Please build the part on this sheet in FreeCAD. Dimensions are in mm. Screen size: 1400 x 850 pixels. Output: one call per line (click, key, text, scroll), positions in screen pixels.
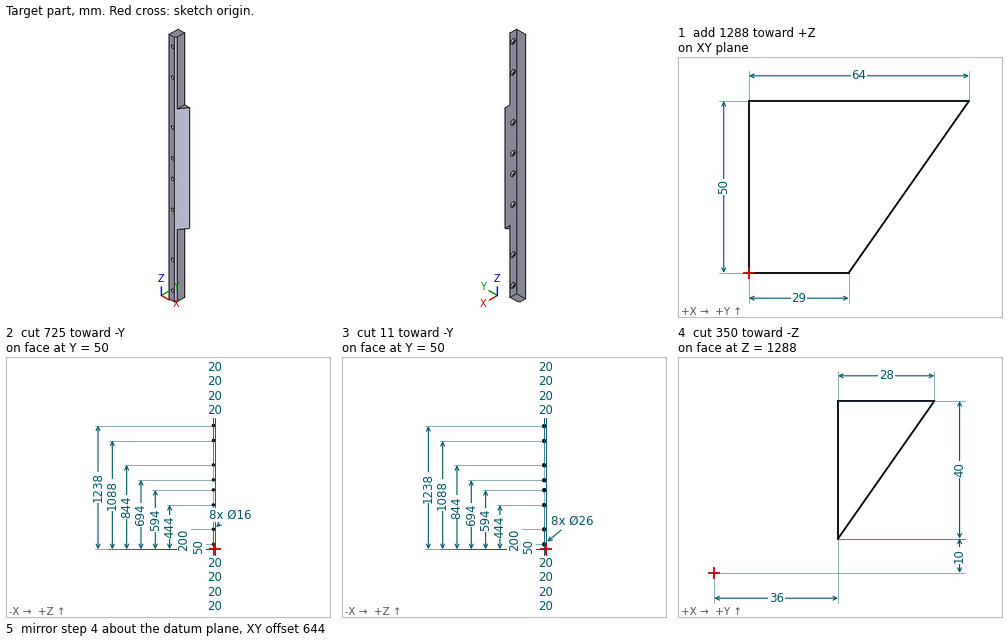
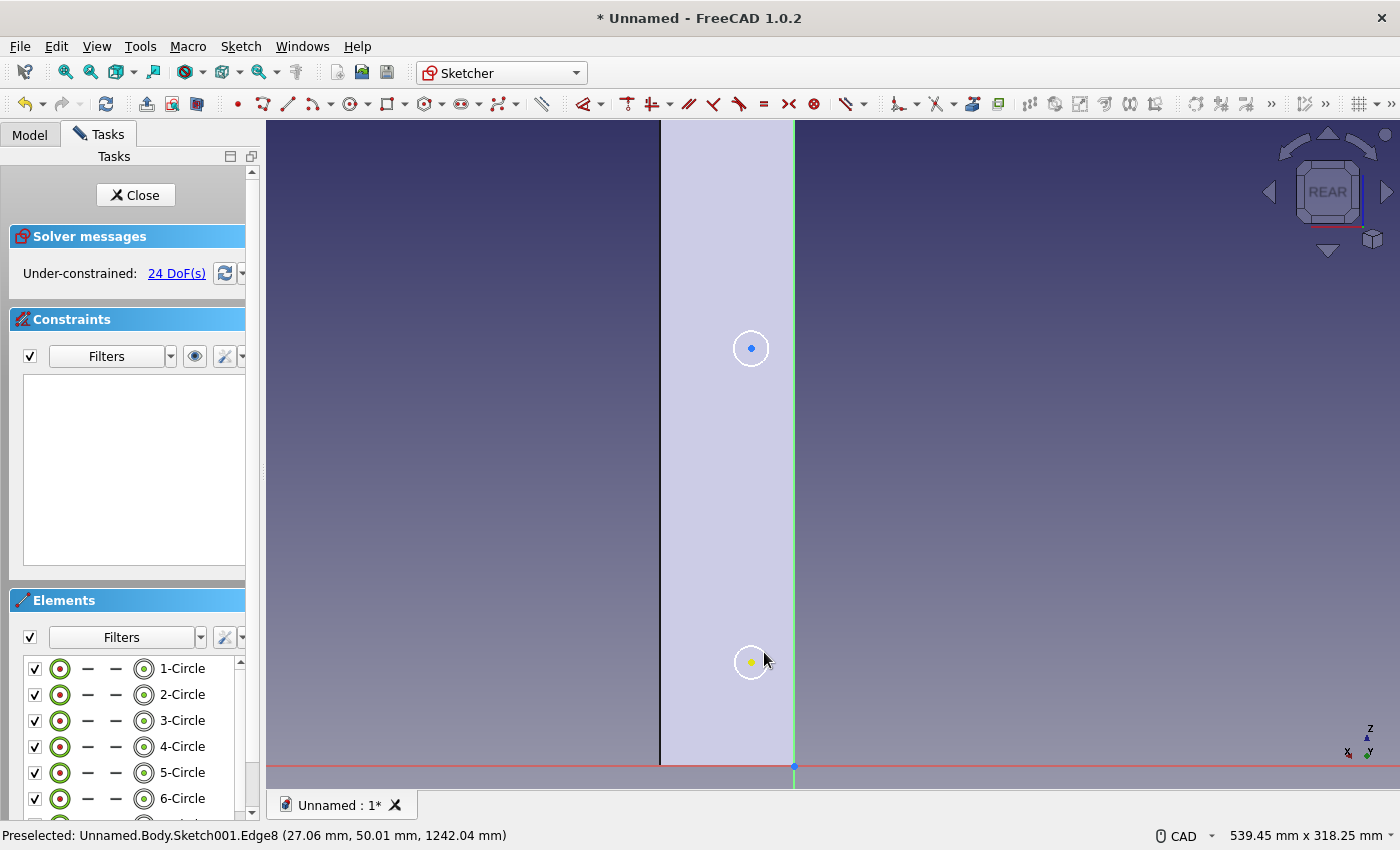
click(763, 651)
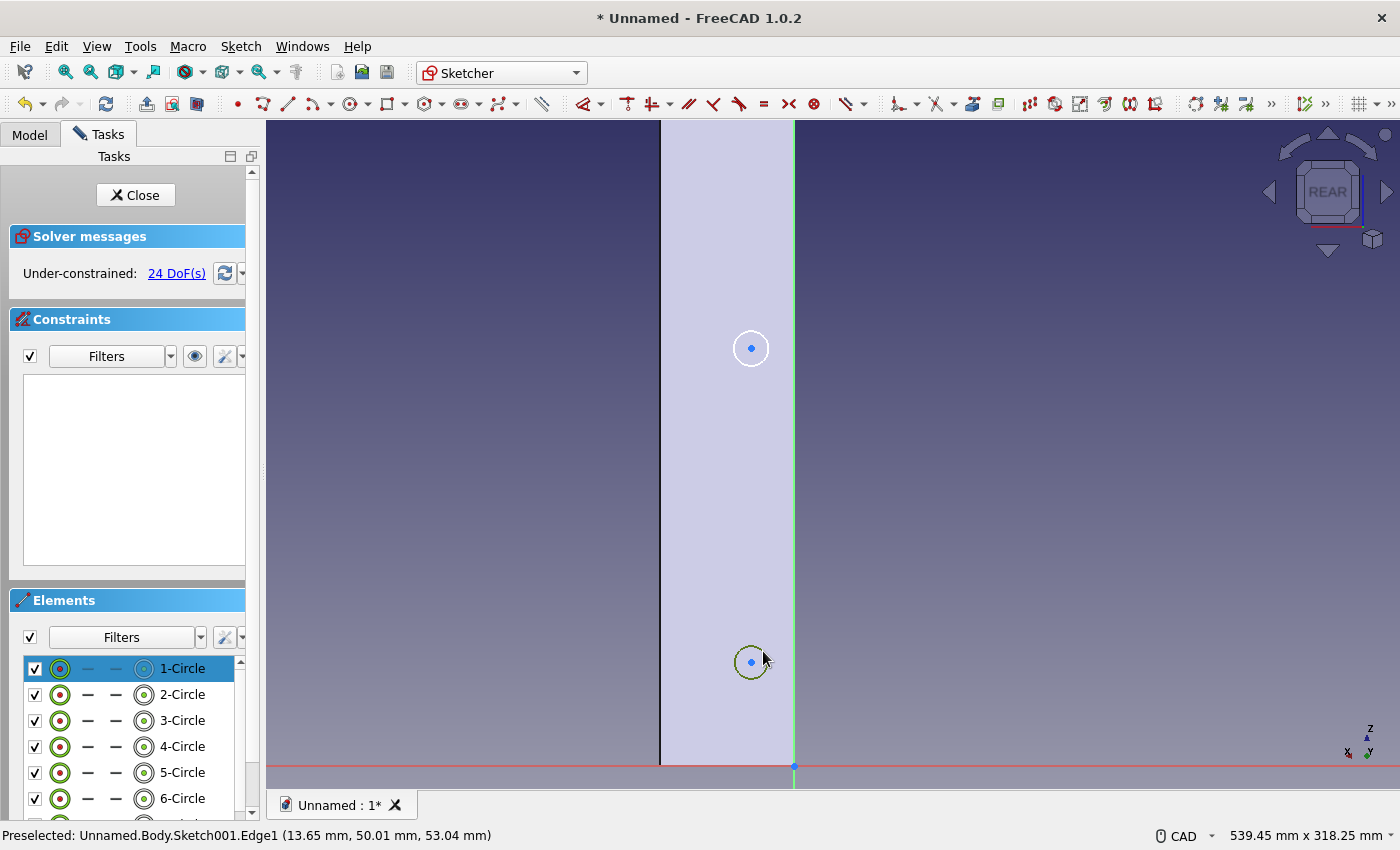
click(763, 336)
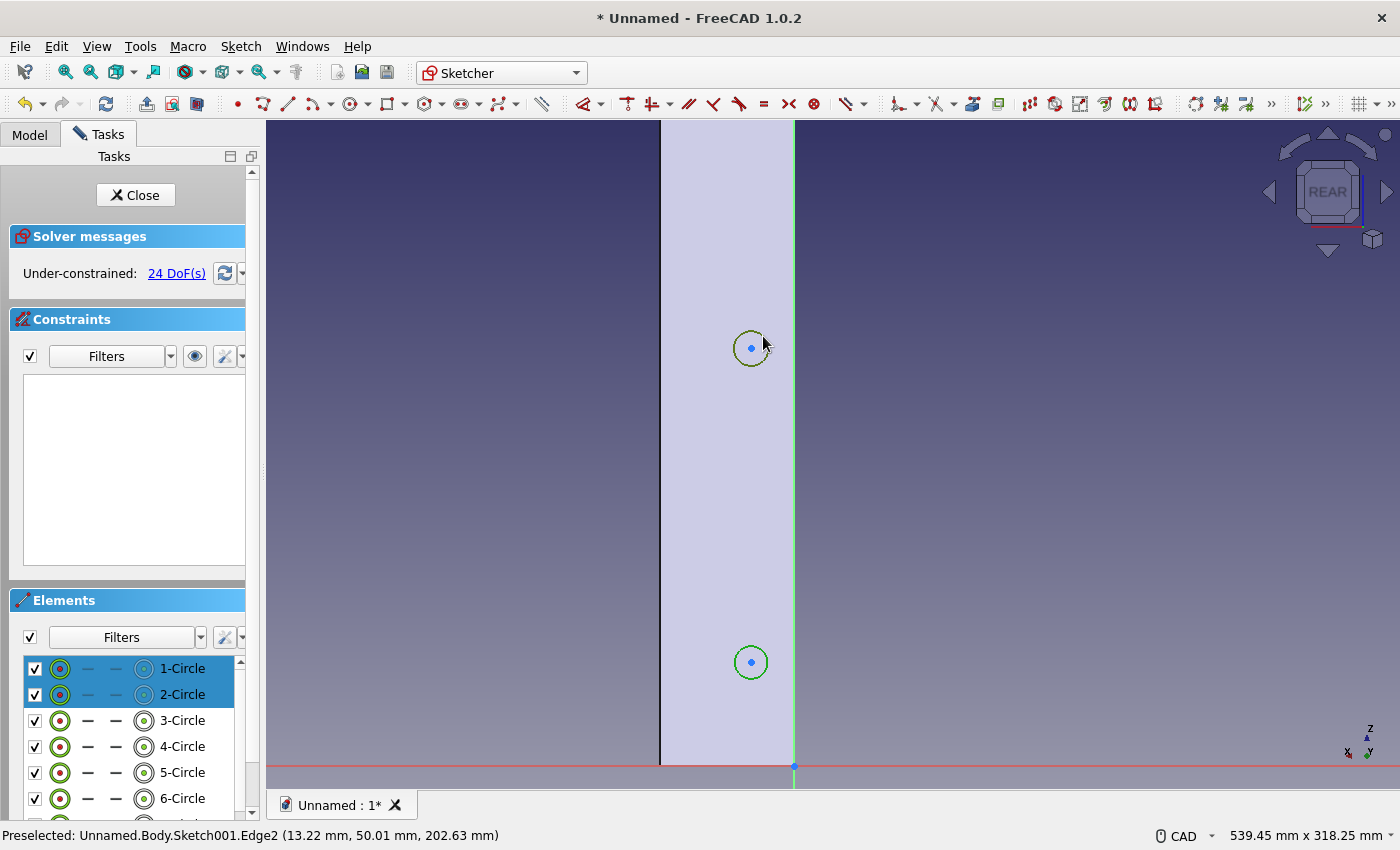
scroll(764, 652, down, 9)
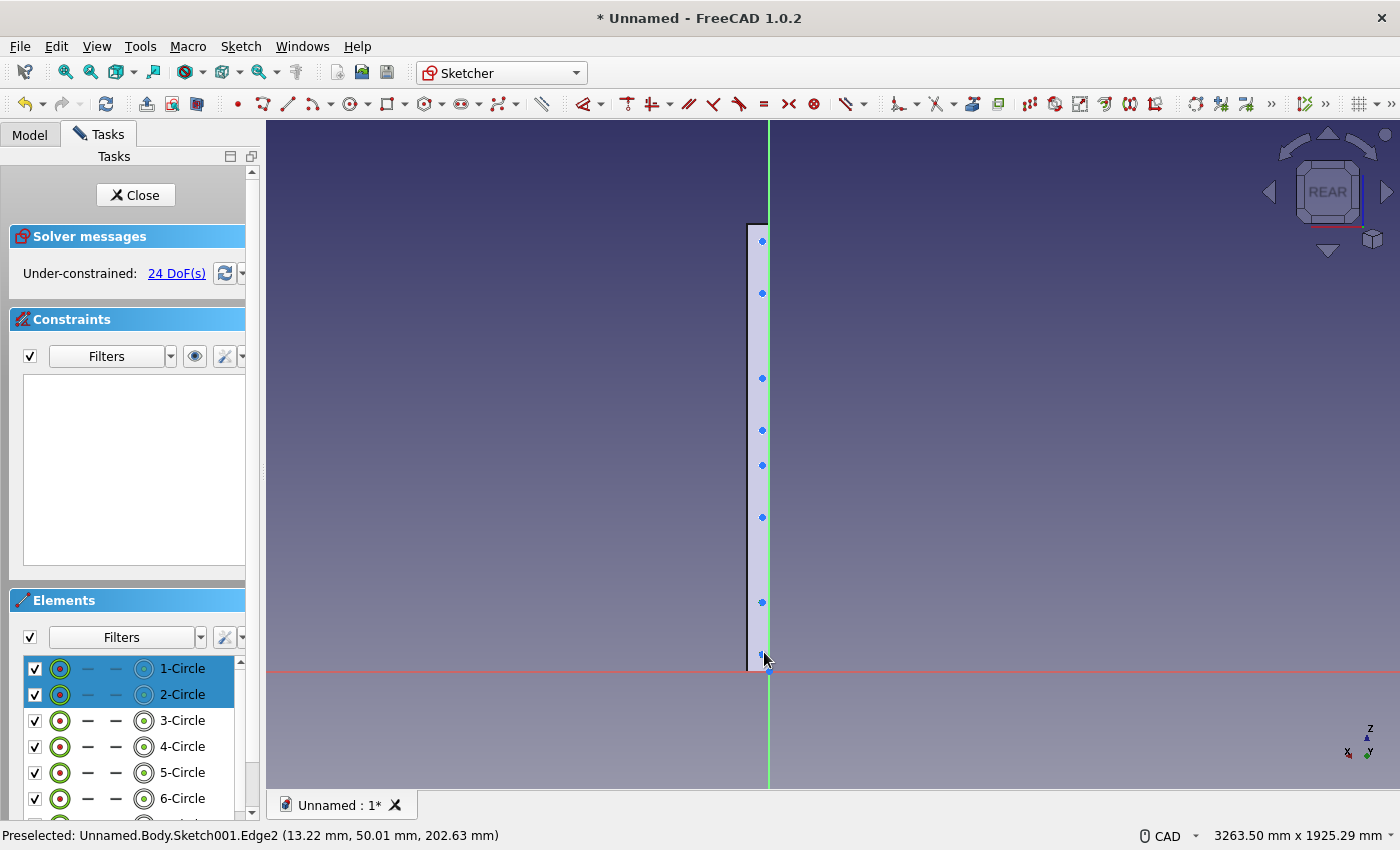
scroll(764, 516, up, 8)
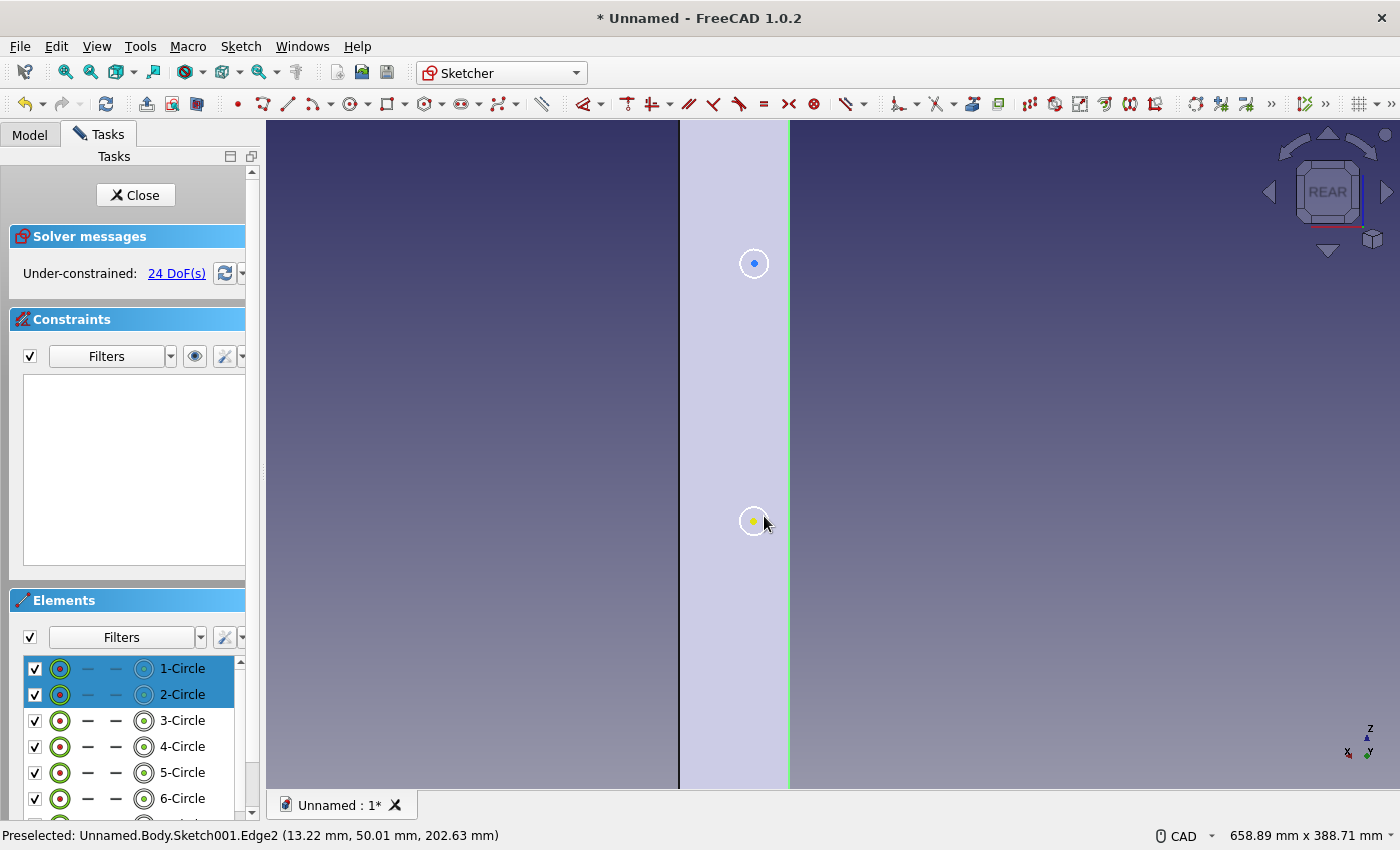
click(764, 511)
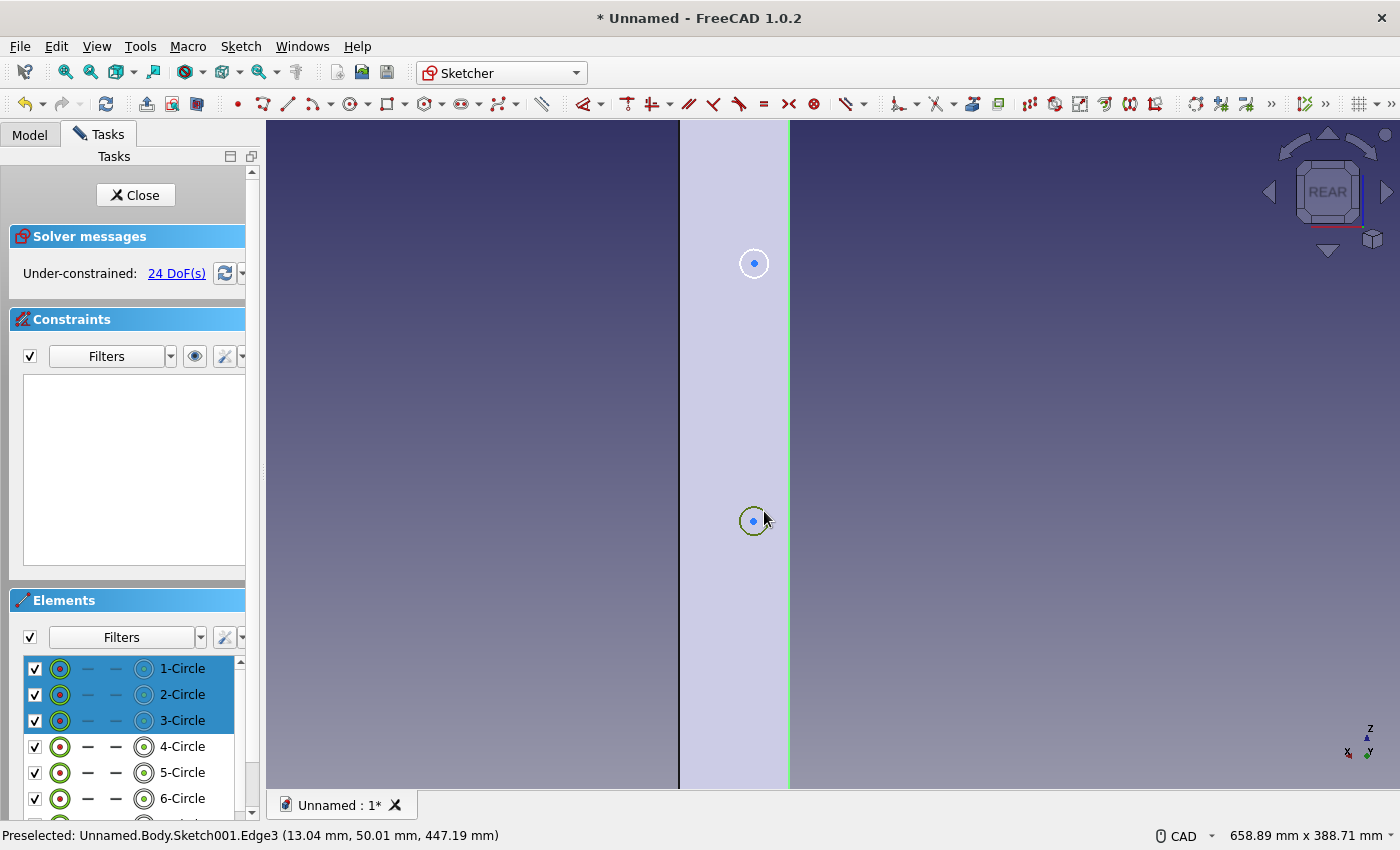
click(764, 254)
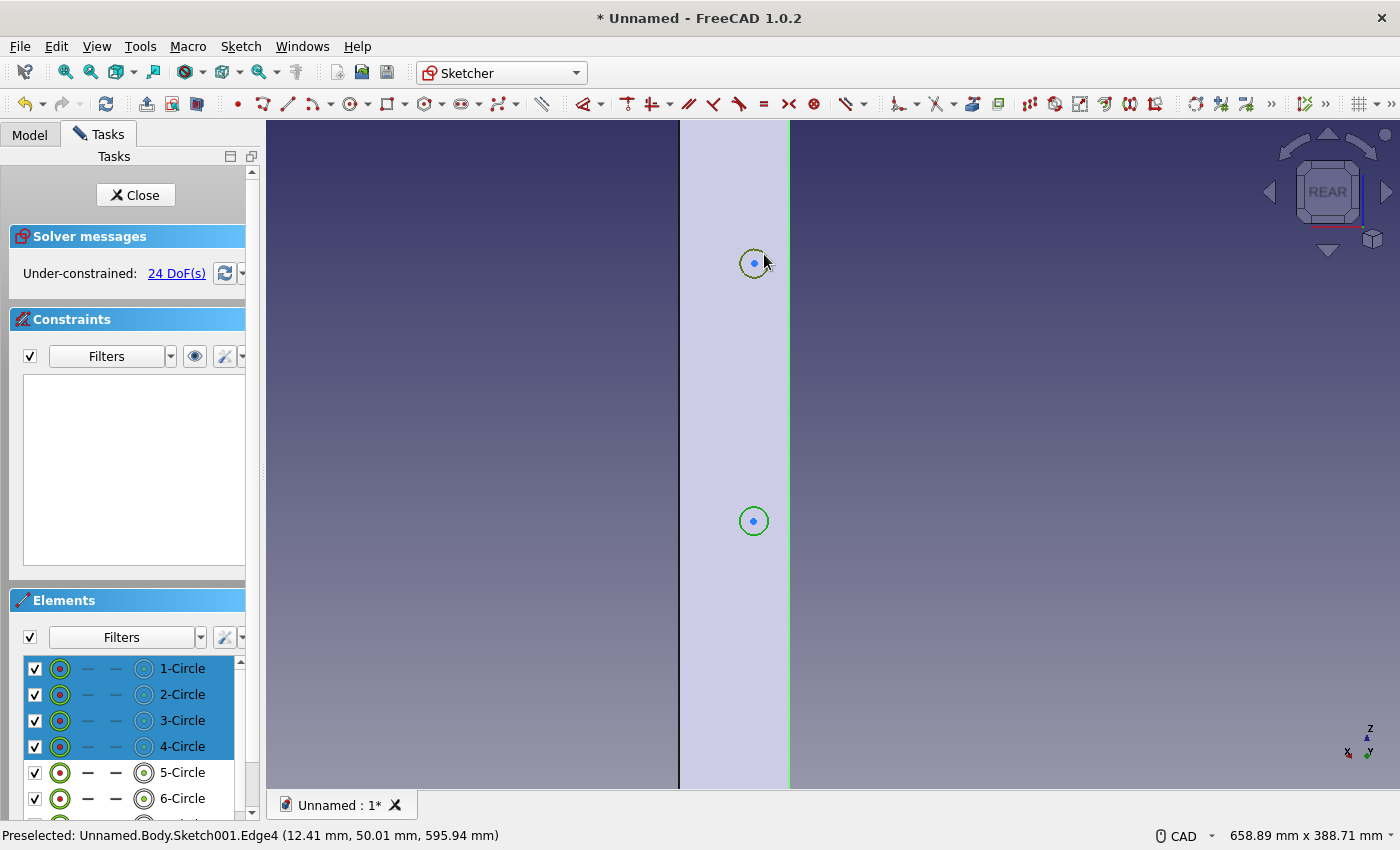
scroll(764, 516, down, 8)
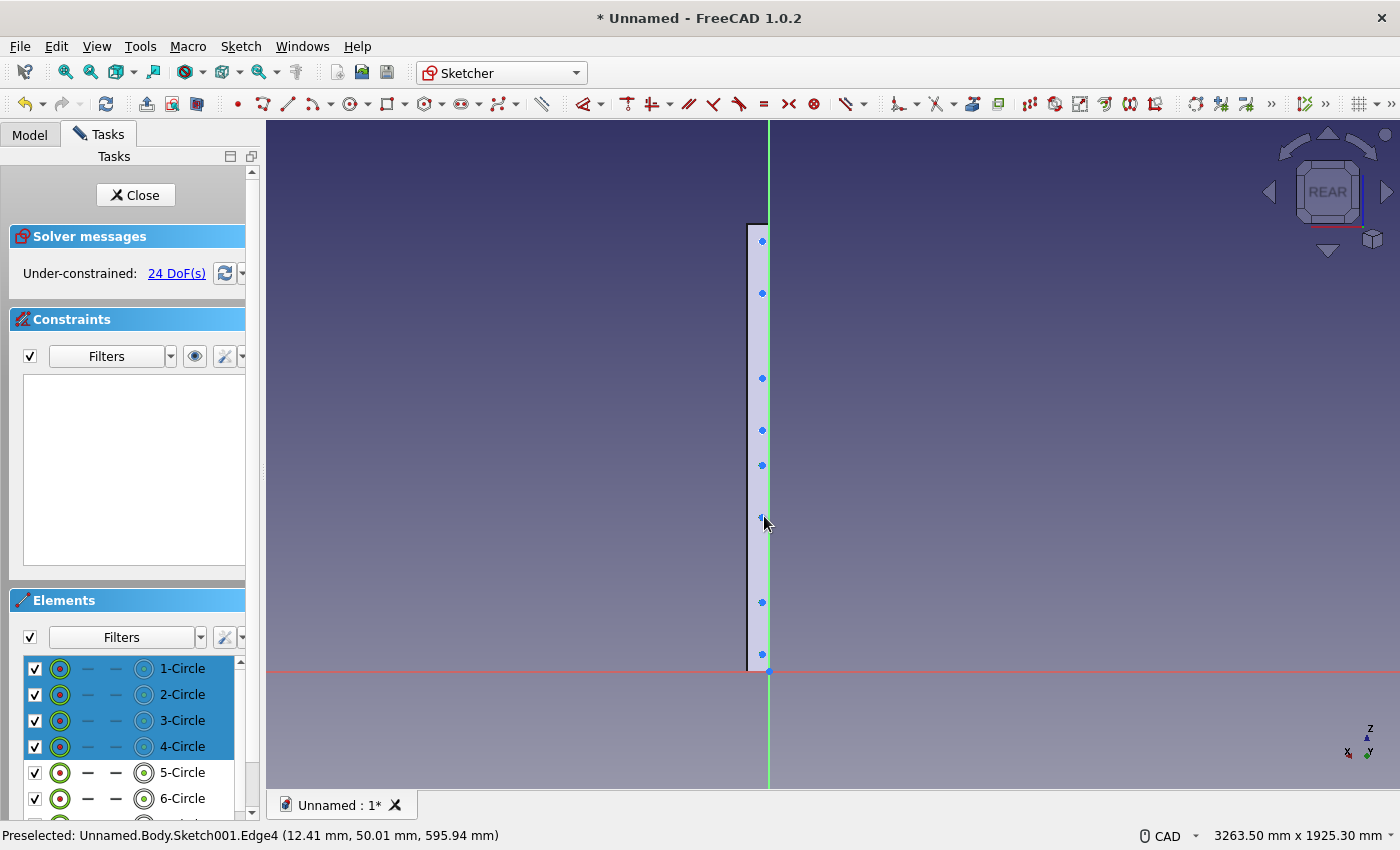
scroll(764, 429, up, 8)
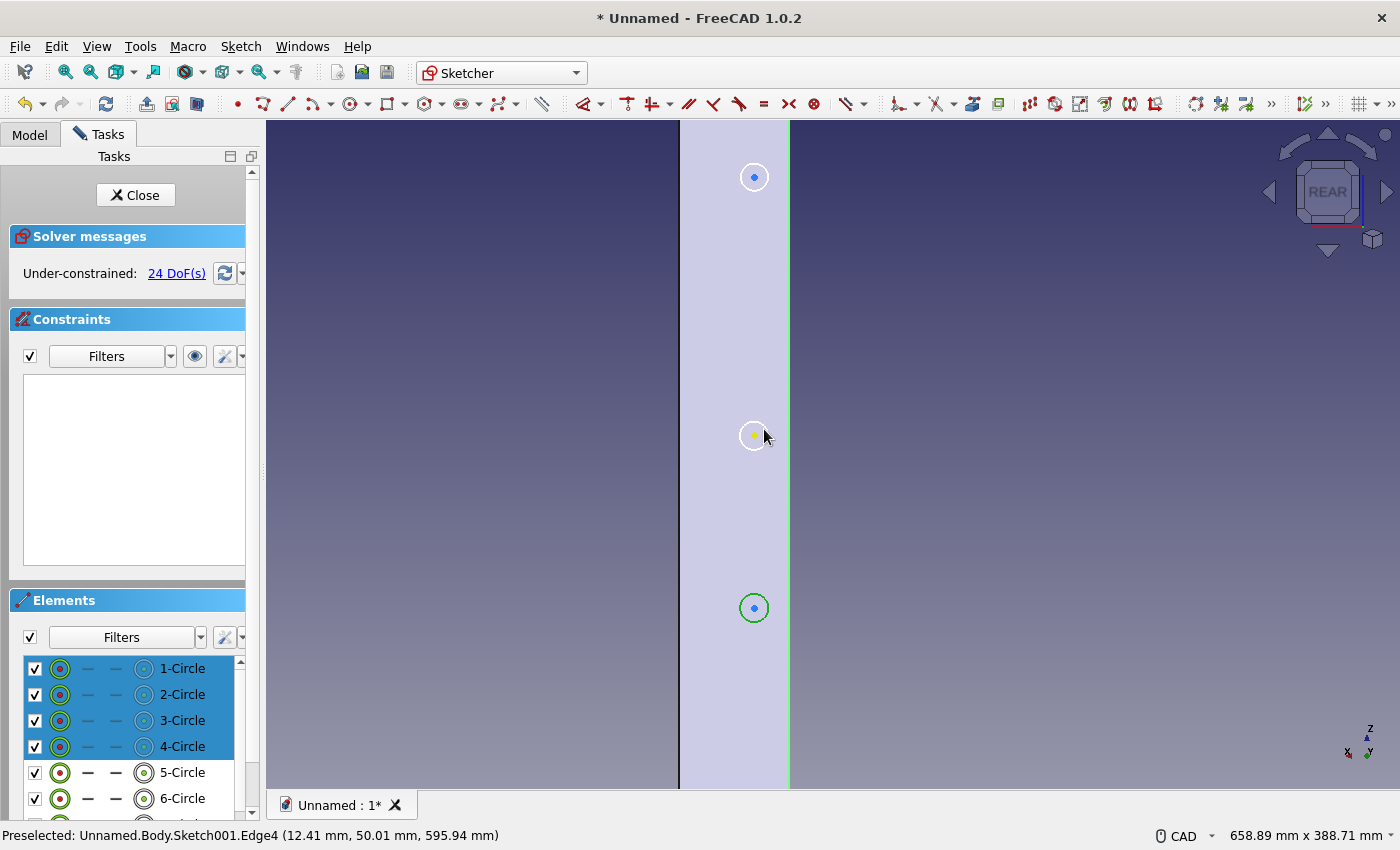
click(764, 426)